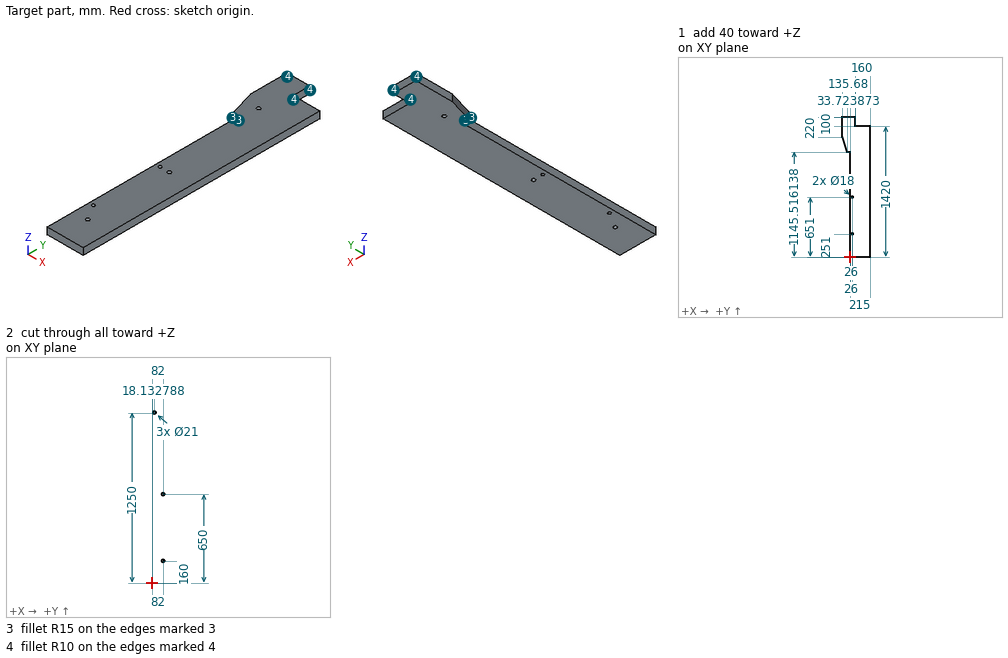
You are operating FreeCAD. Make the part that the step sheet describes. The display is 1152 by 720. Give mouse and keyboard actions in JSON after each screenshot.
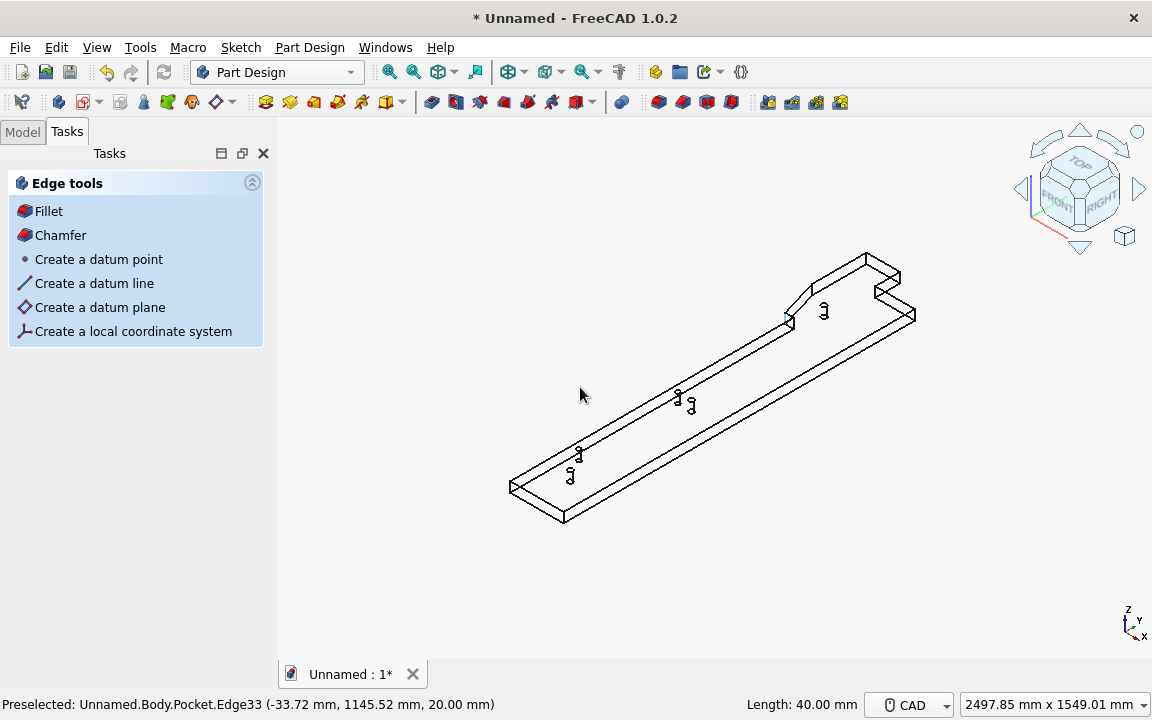
{"action": "left_click", "coordinate": [794, 325], "text": "ctrl"}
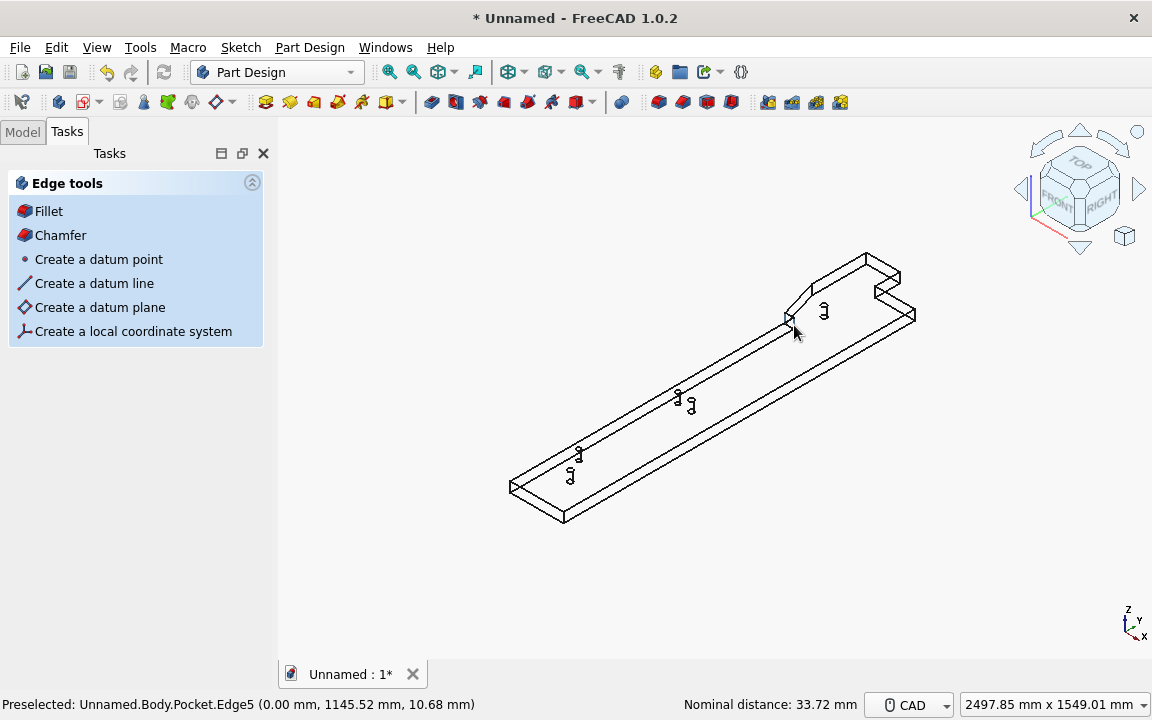
{"action": "key", "text": "v 1"}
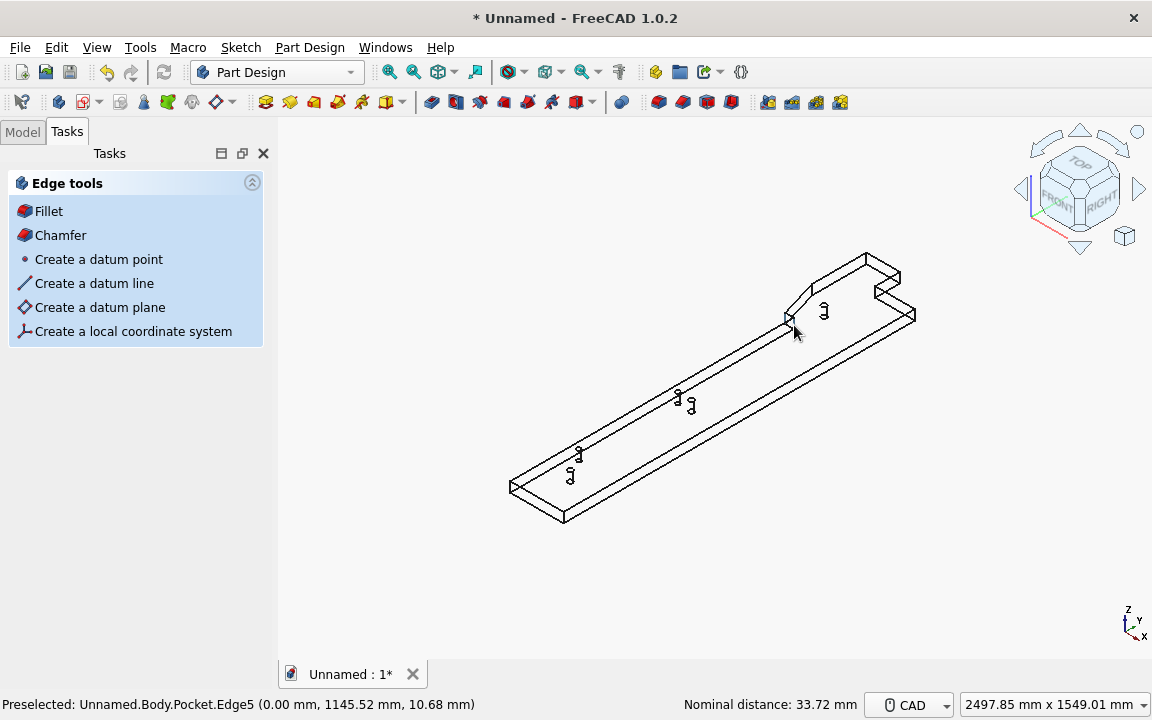
{"action": "left_click", "coordinate": [660, 102]}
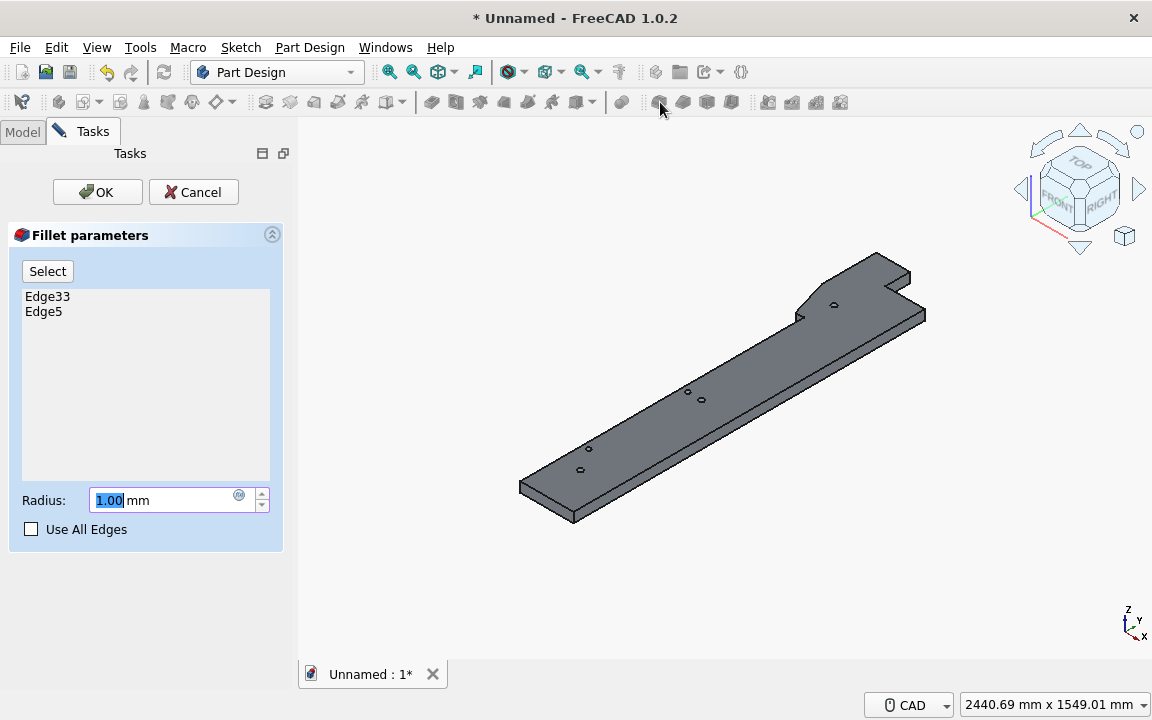
{"action": "type", "text": "15"}
{"action": "key", "text": "Tab"}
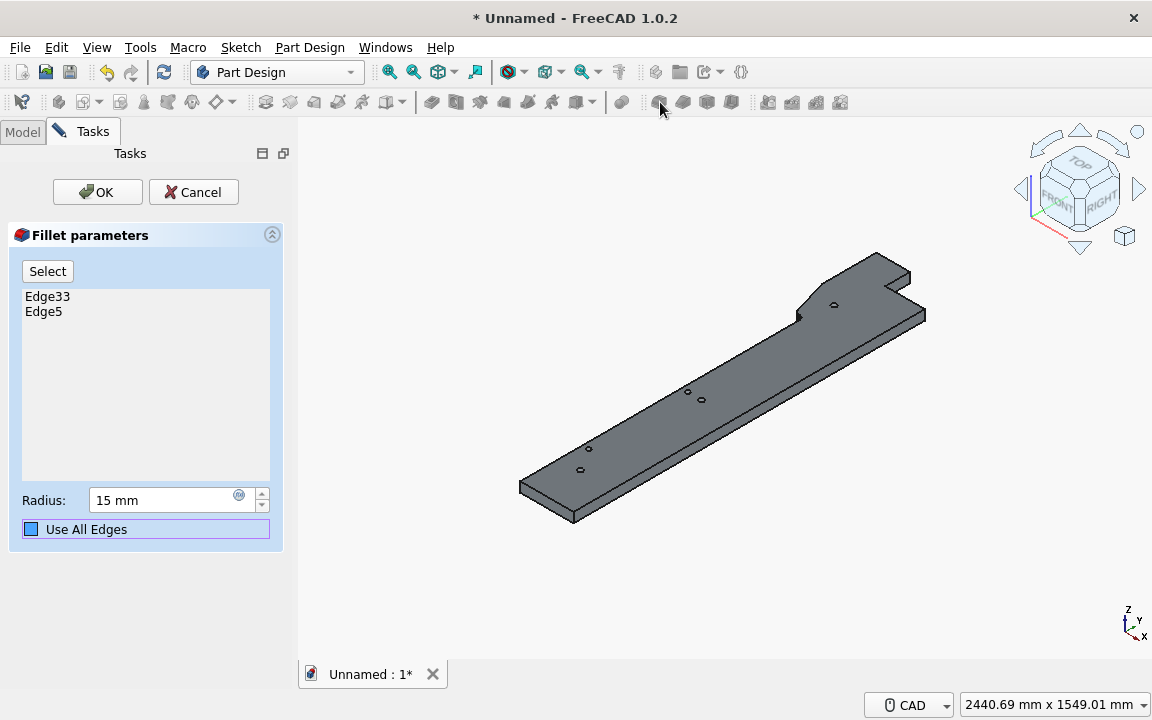
{"action": "left_click", "coordinate": [98, 192]}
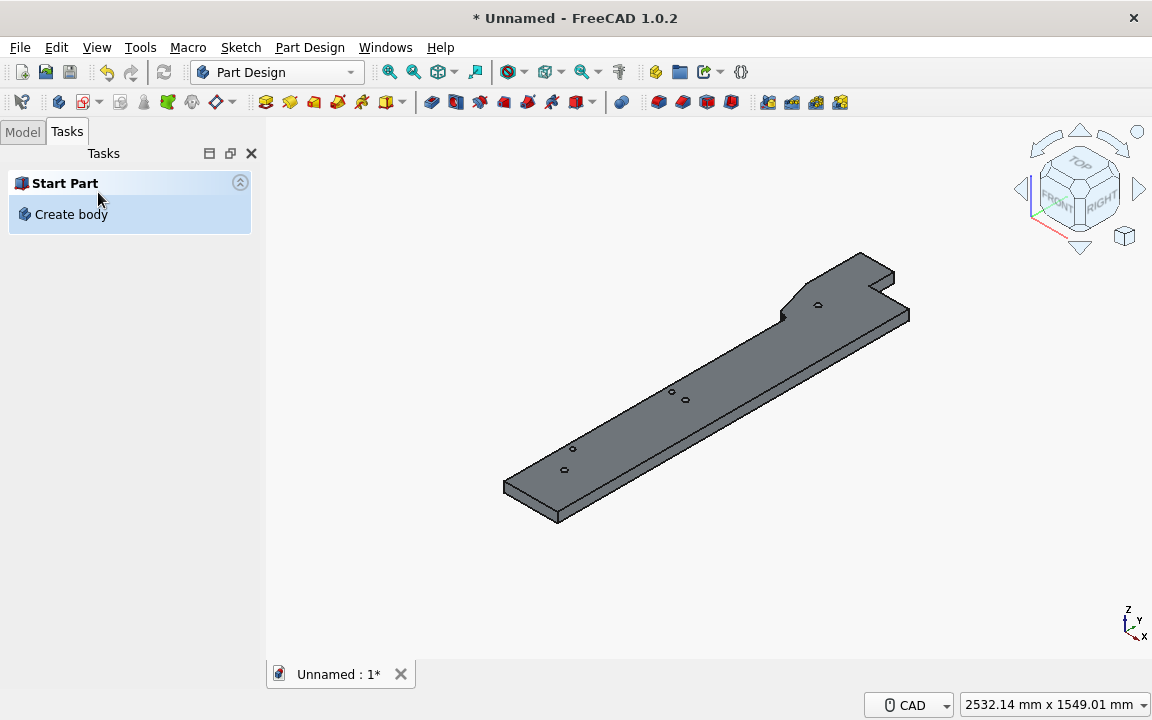
{"action": "scroll", "coordinate": [860, 257], "scroll_direction": "up", "scroll_amount": 6}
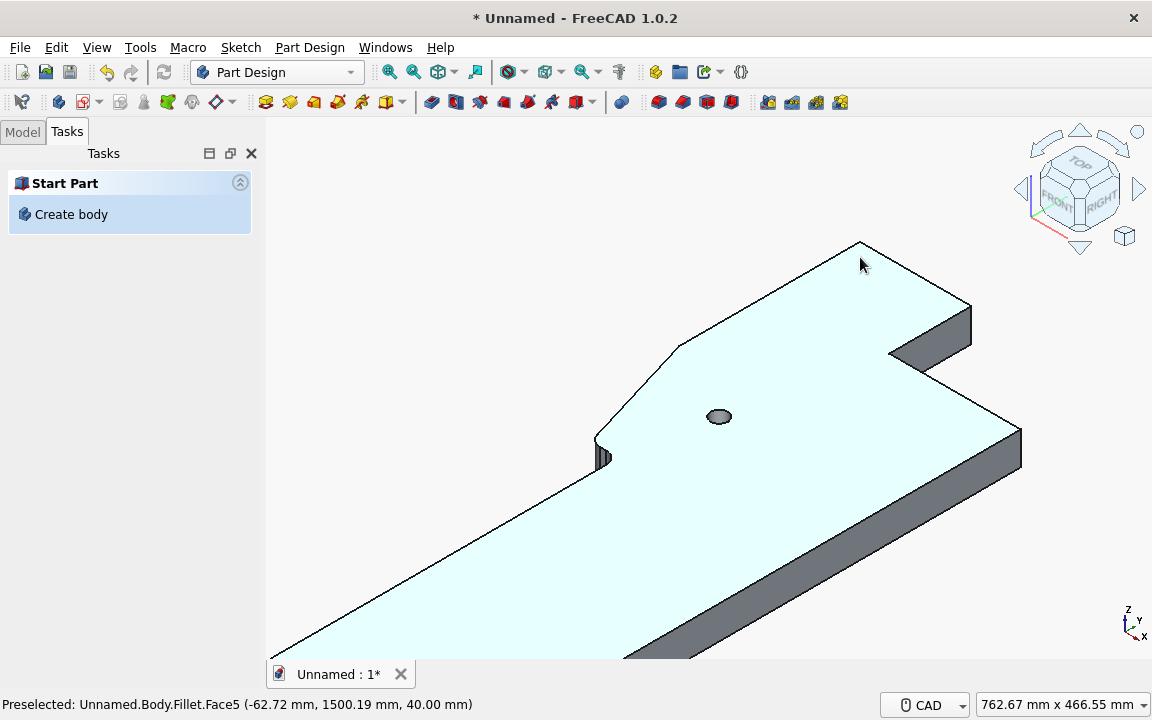
{"action": "left_click", "coordinate": [390, 72]}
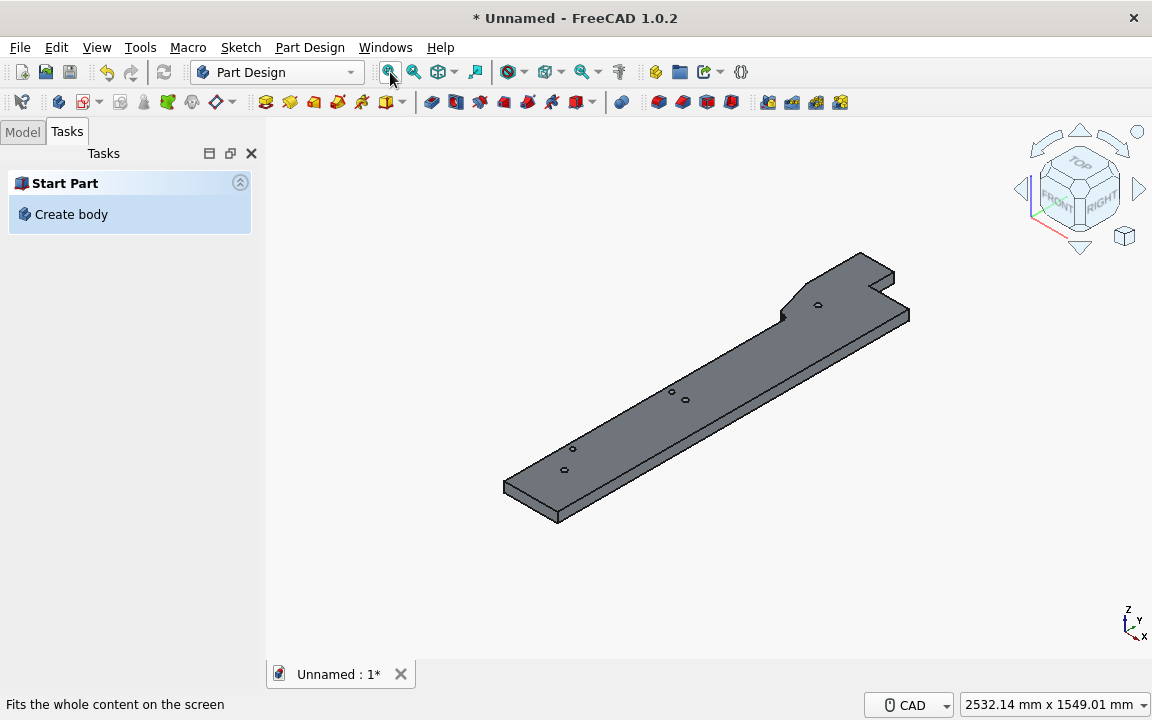
{"action": "key", "text": "2"}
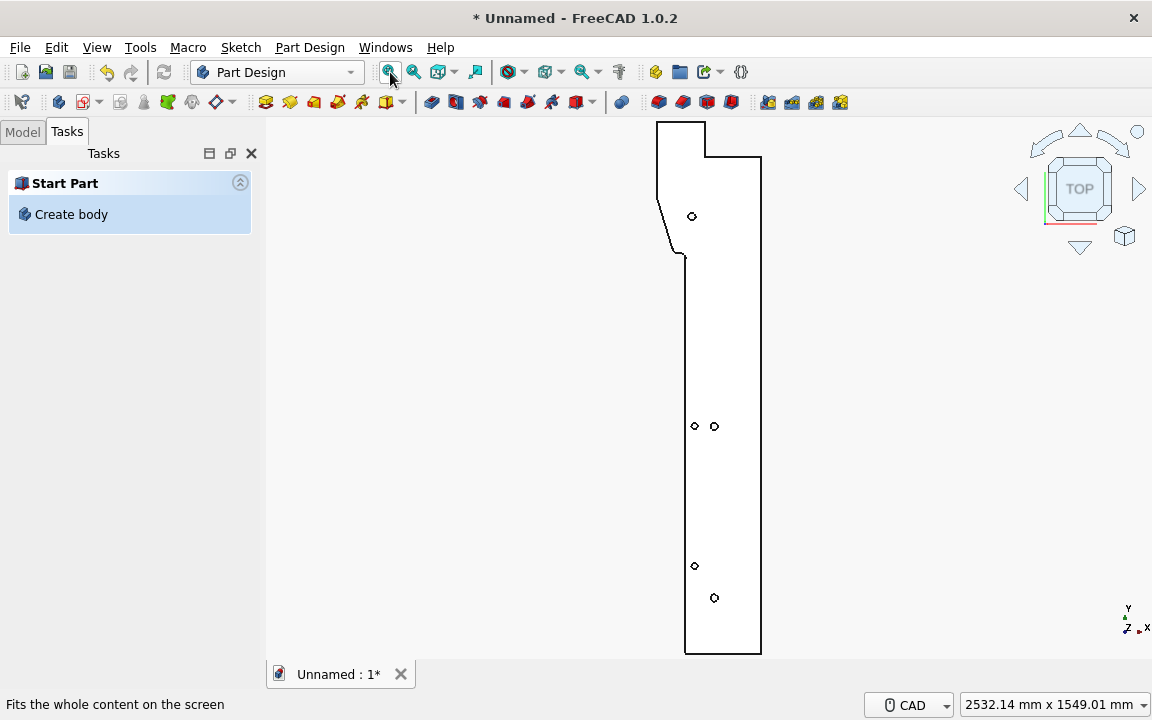
{"action": "key", "text": "0"}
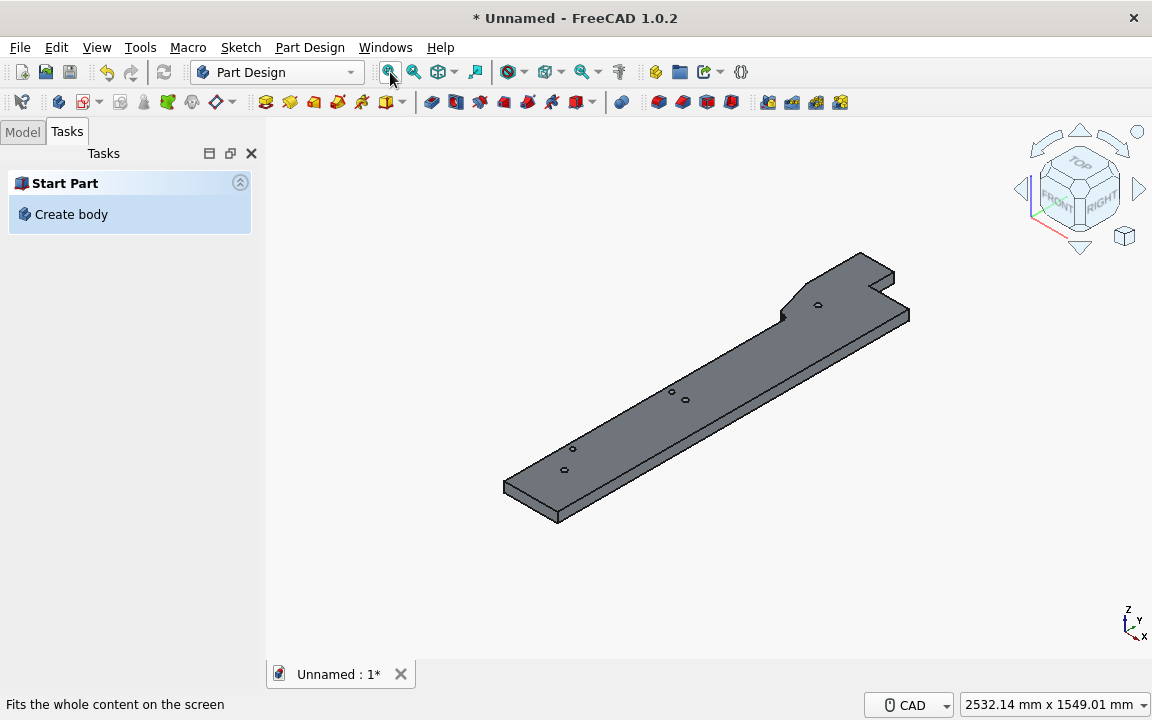
{"action": "scroll", "coordinate": [860, 257], "scroll_direction": "up", "scroll_amount": 6}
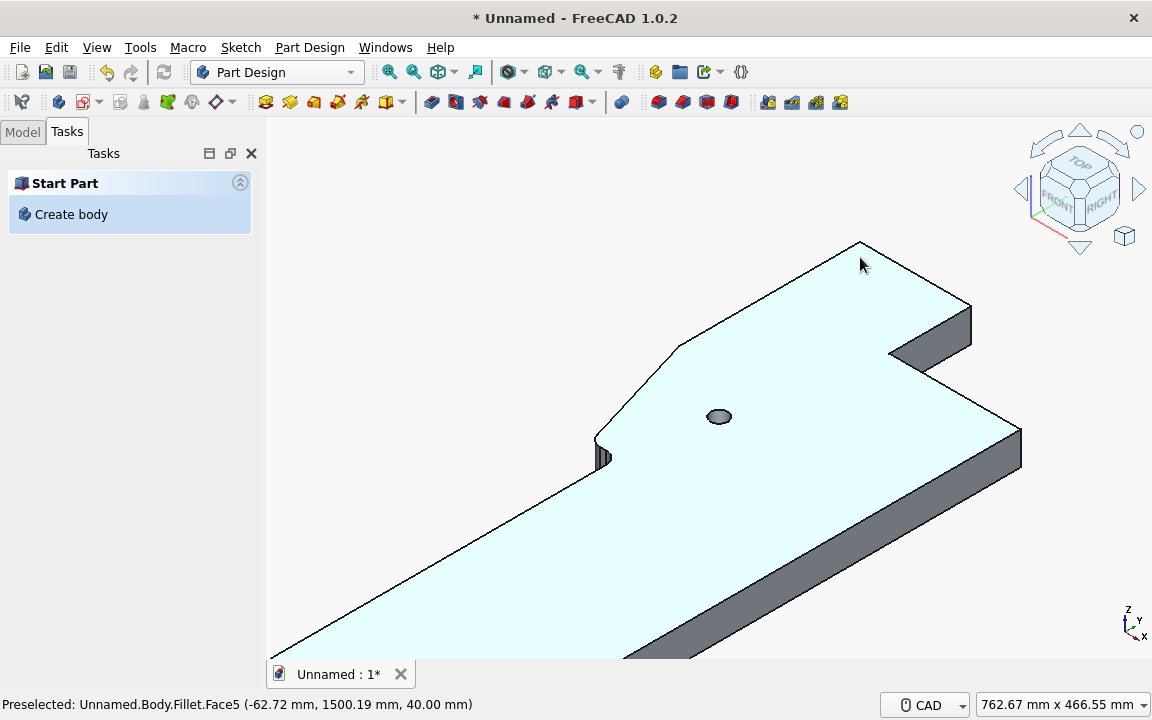
{"action": "key", "text": "v f"}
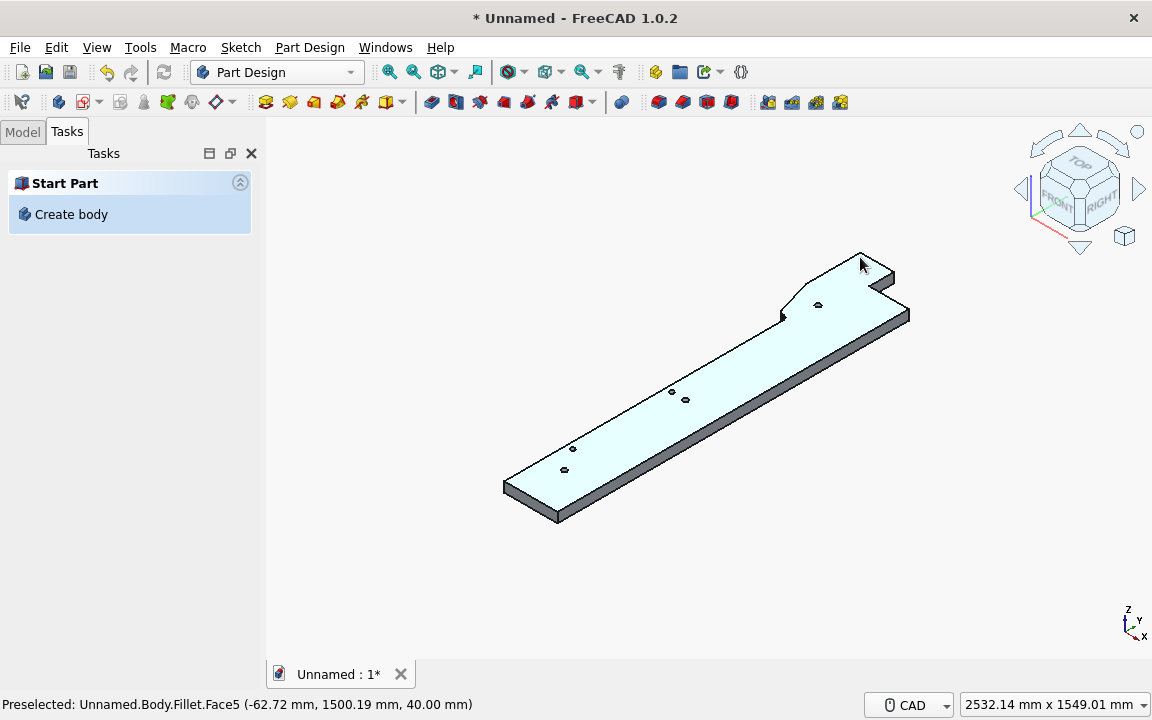
{"action": "key", "text": "1"}